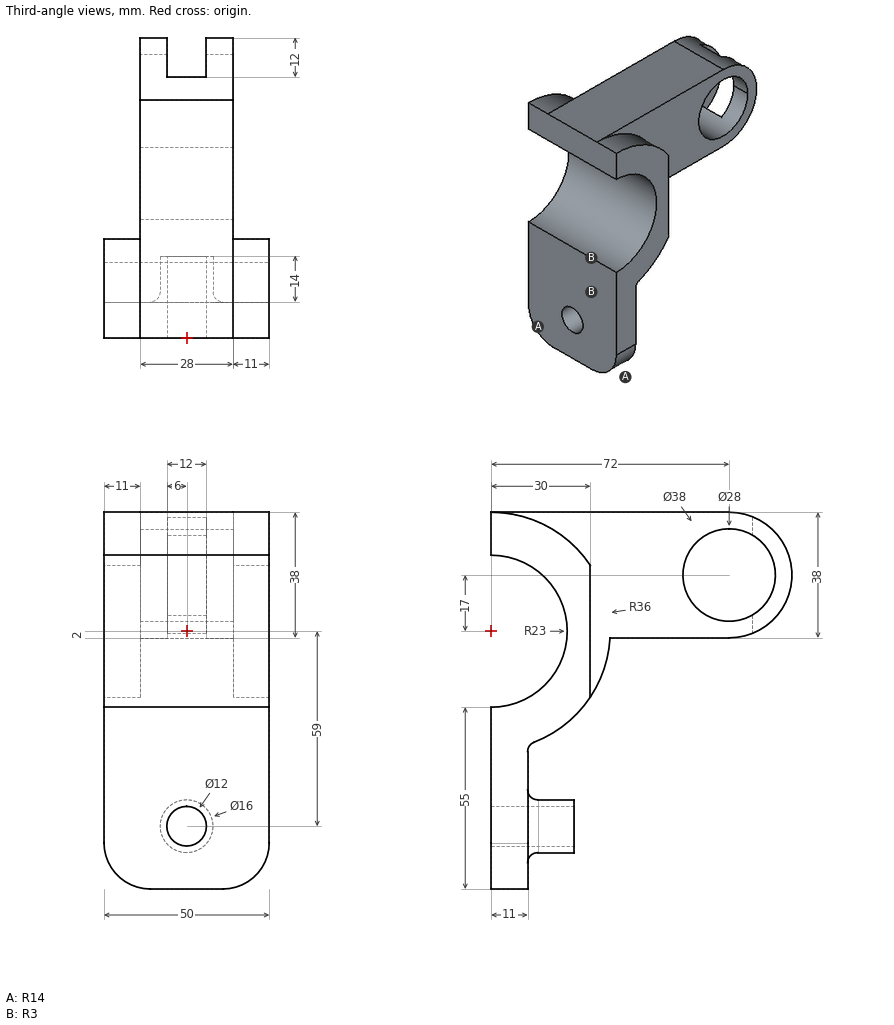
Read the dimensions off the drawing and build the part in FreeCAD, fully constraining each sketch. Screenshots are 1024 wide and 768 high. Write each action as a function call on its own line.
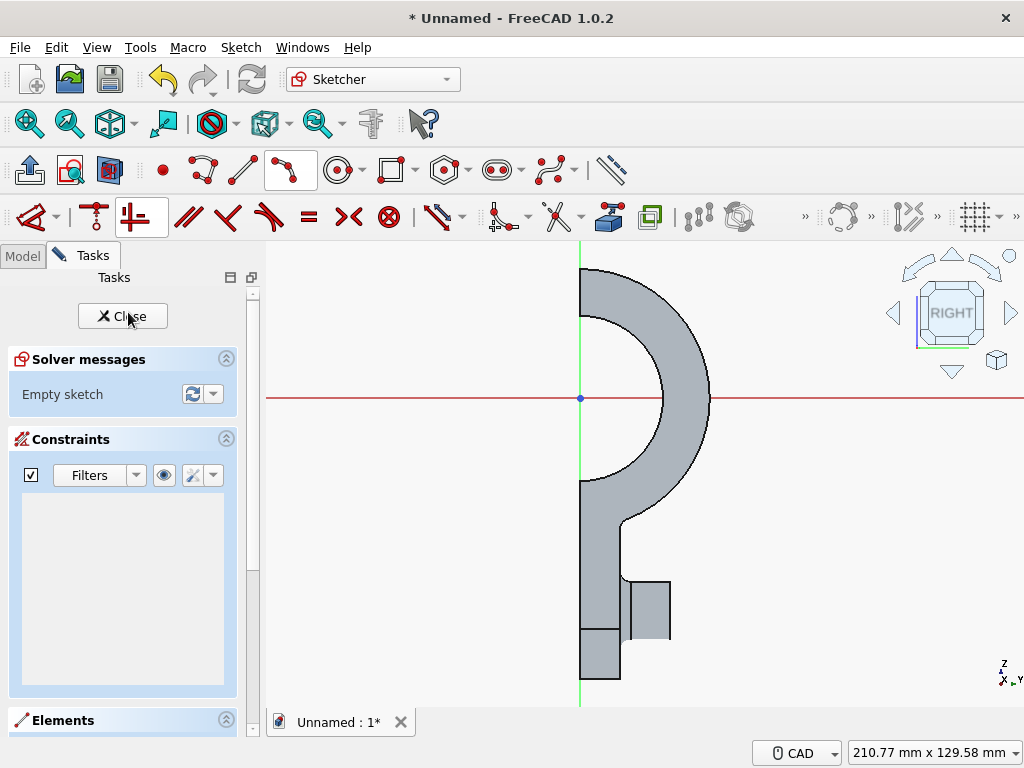
click(110, 170)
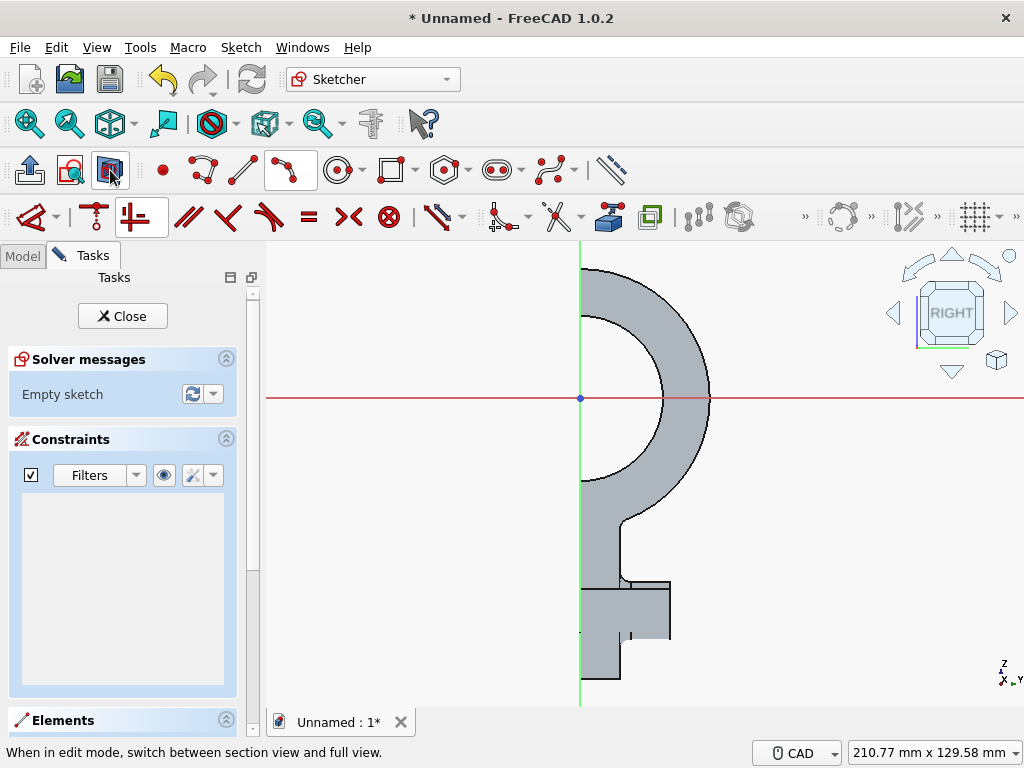
scroll(294, 679, down, 1)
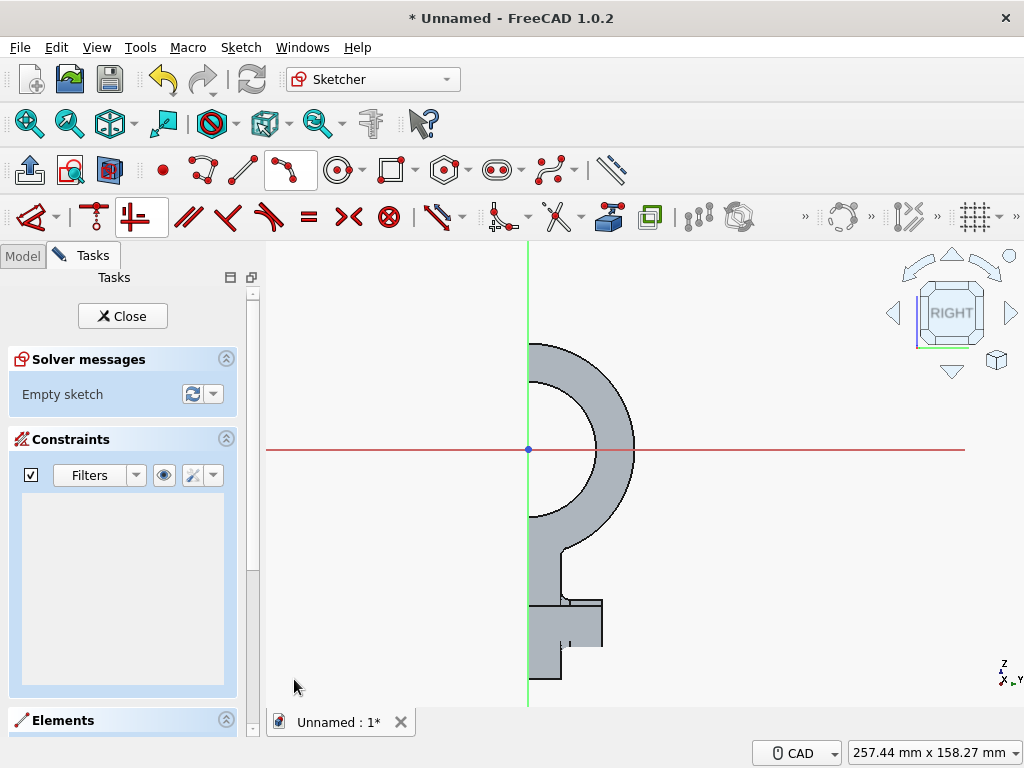
scroll(705, 309, up, 3)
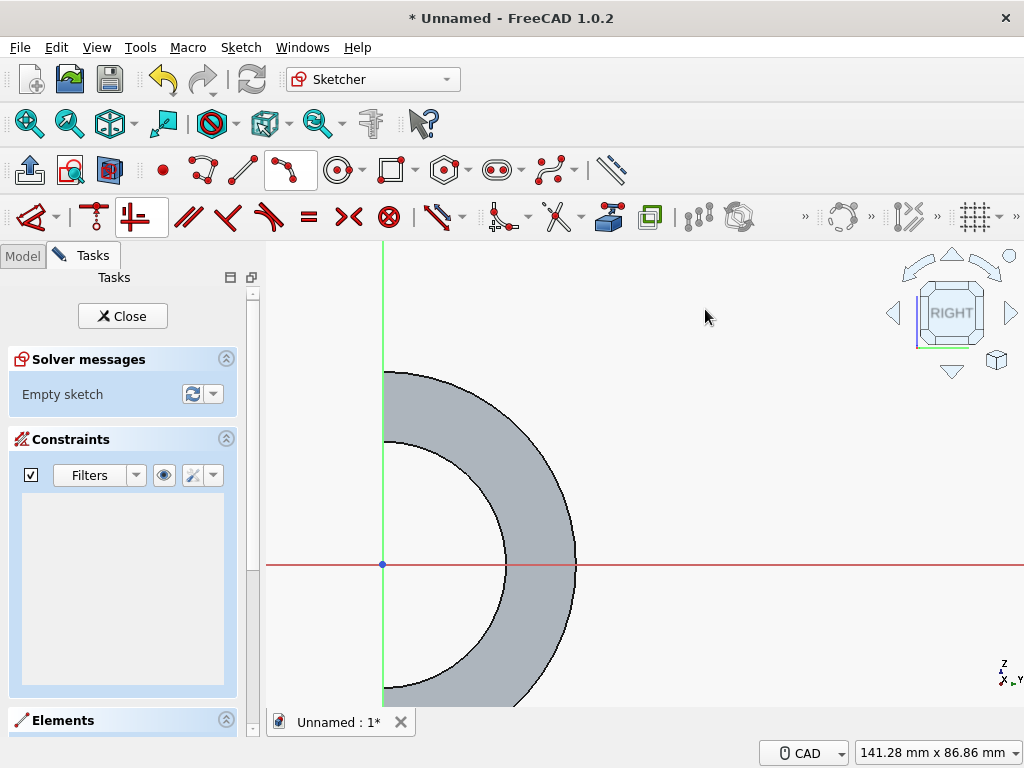
click(204, 170)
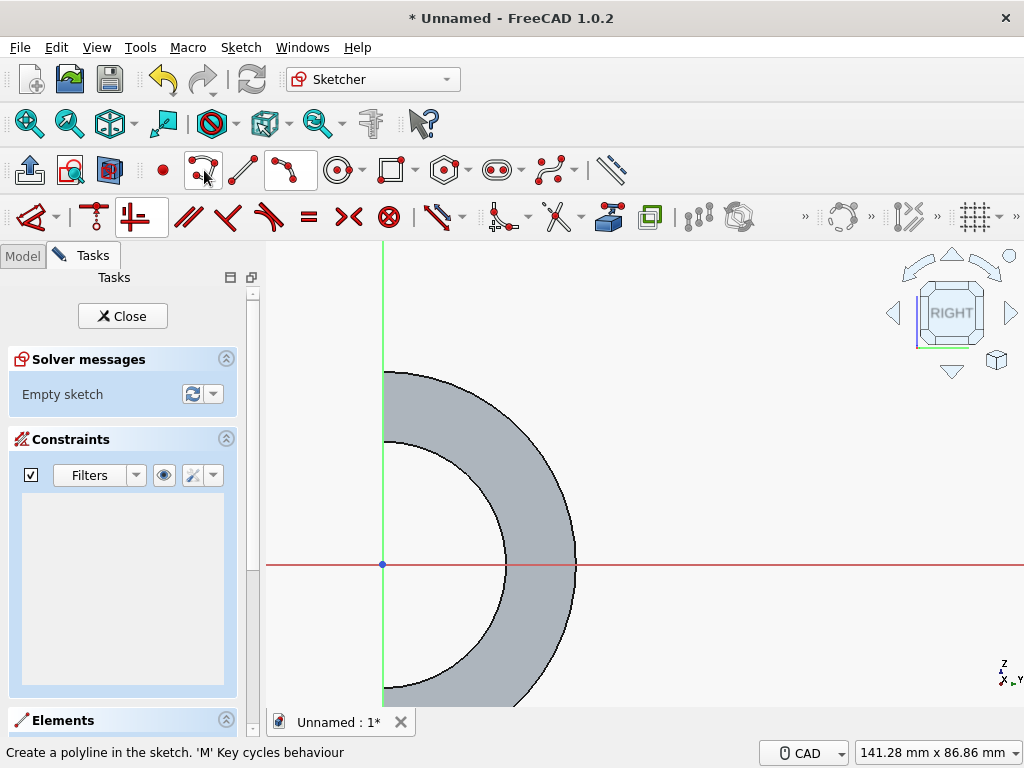
scroll(576, 576, up, 2)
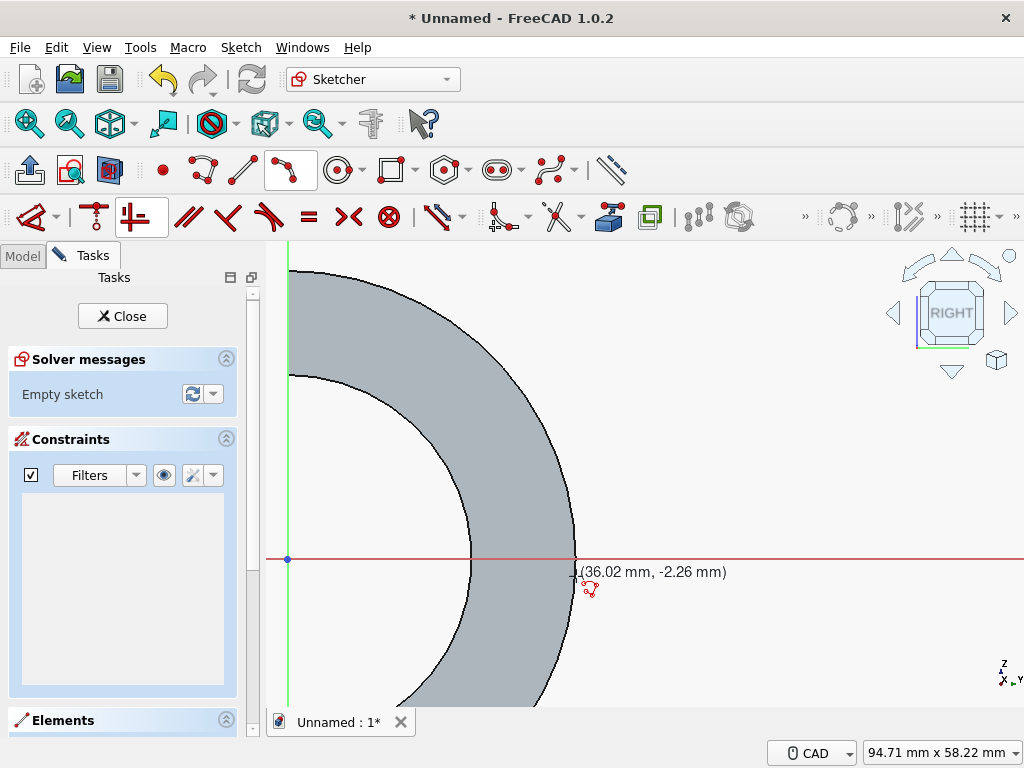
click(575, 575)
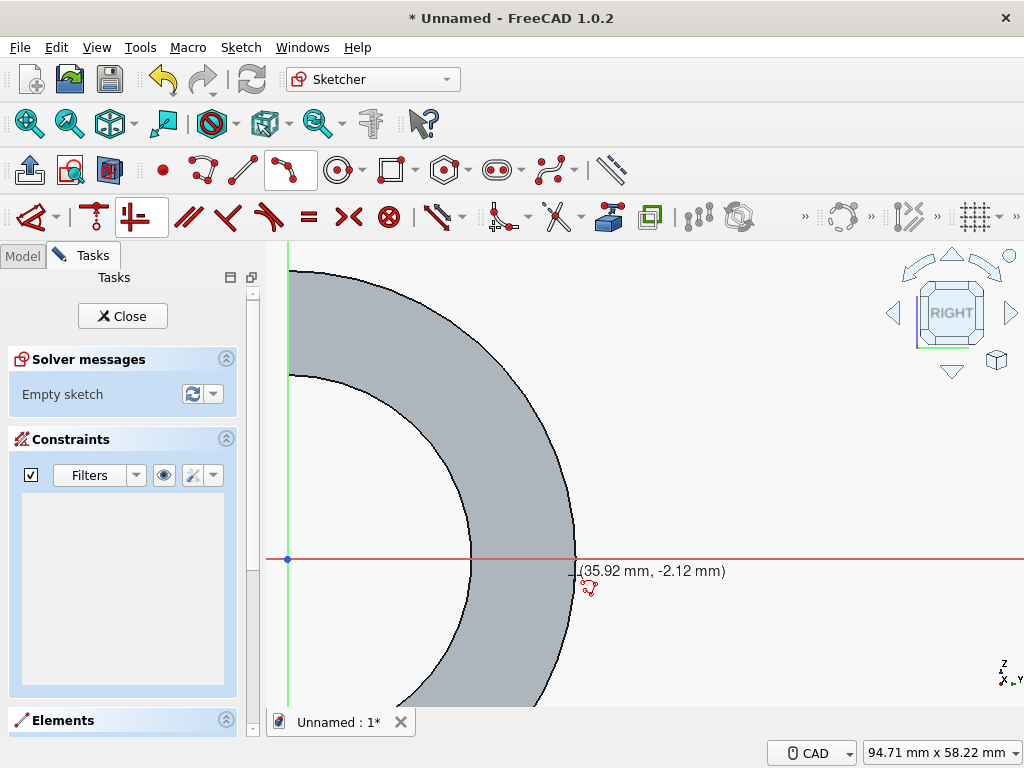
scroll(578, 578, down, 2)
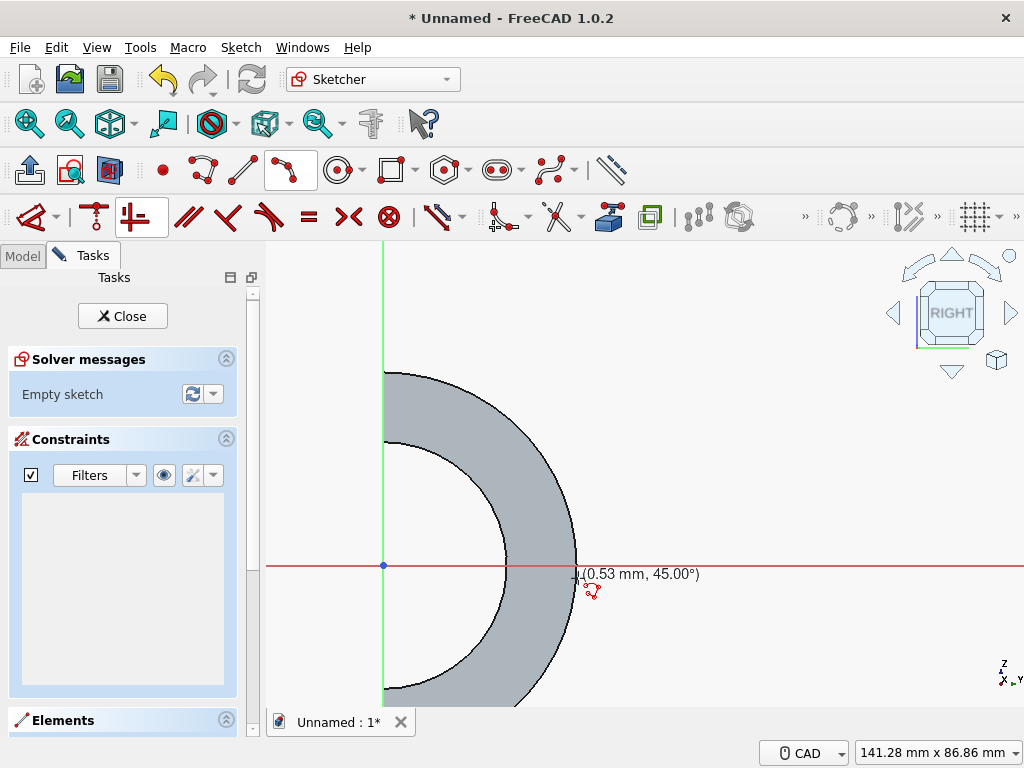
scroll(770, 576, up, 2)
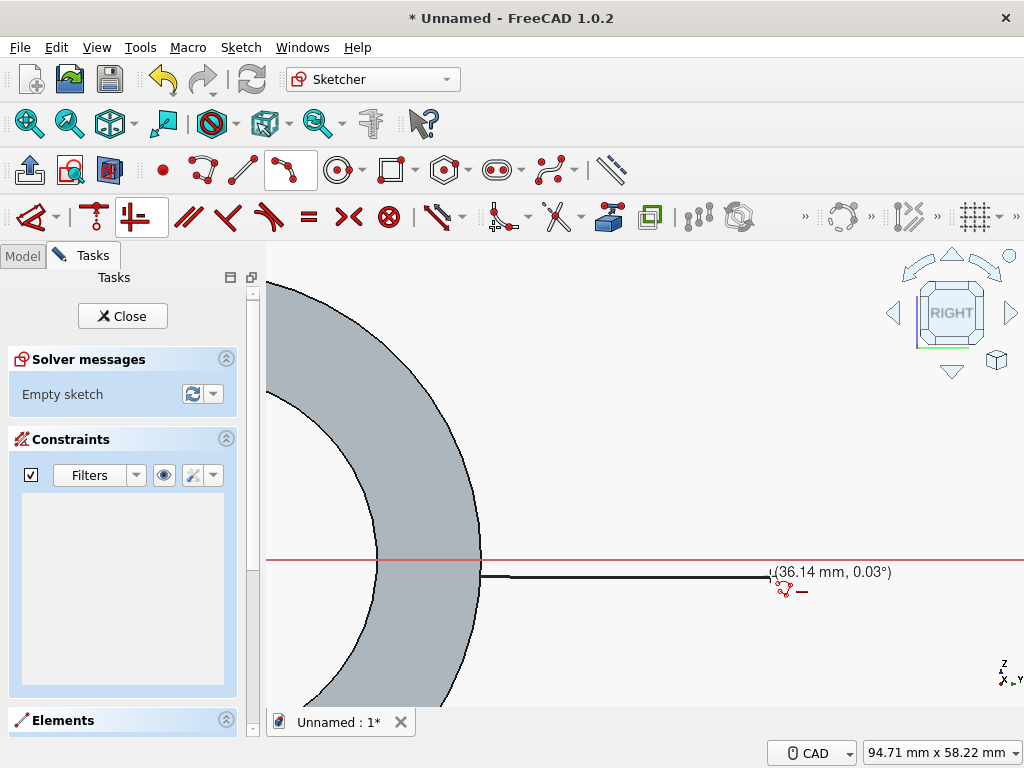
click(769, 576)
click(769, 272)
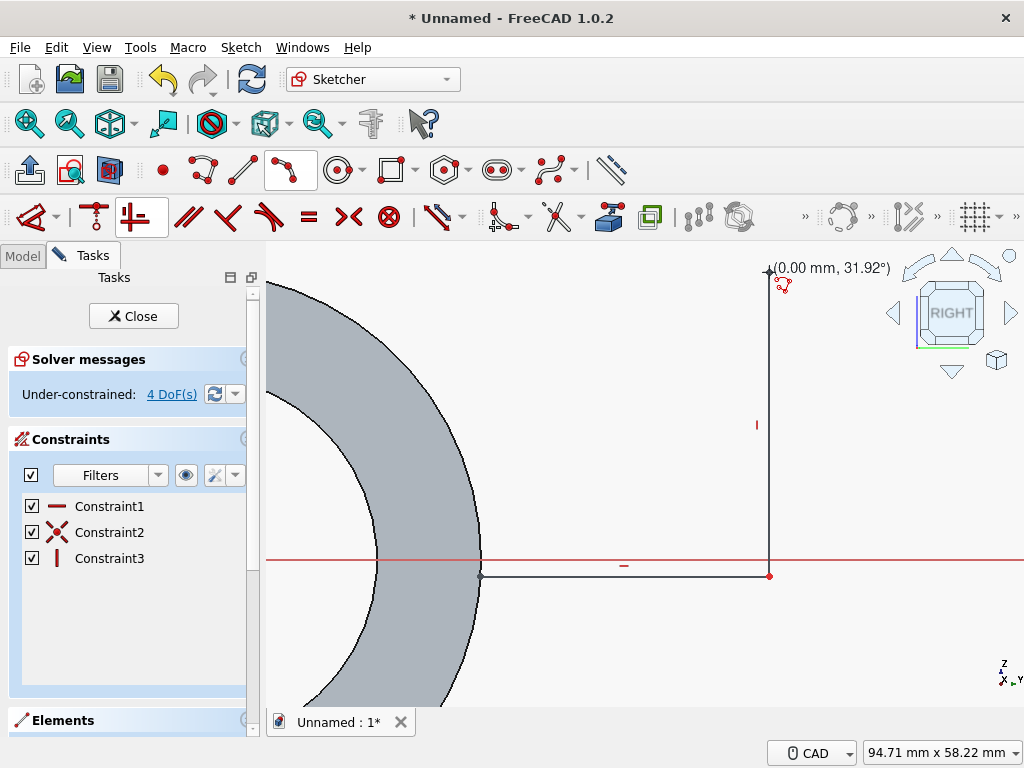
scroll(770, 576, down, 2)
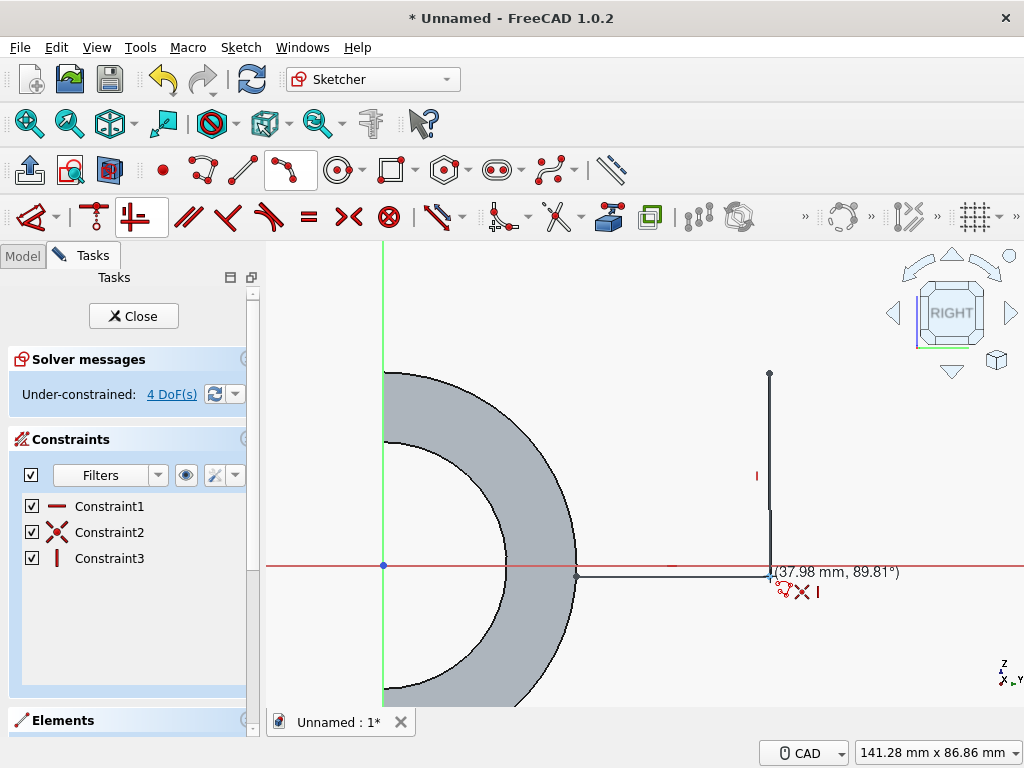
click(383, 372)
right_click(383, 372)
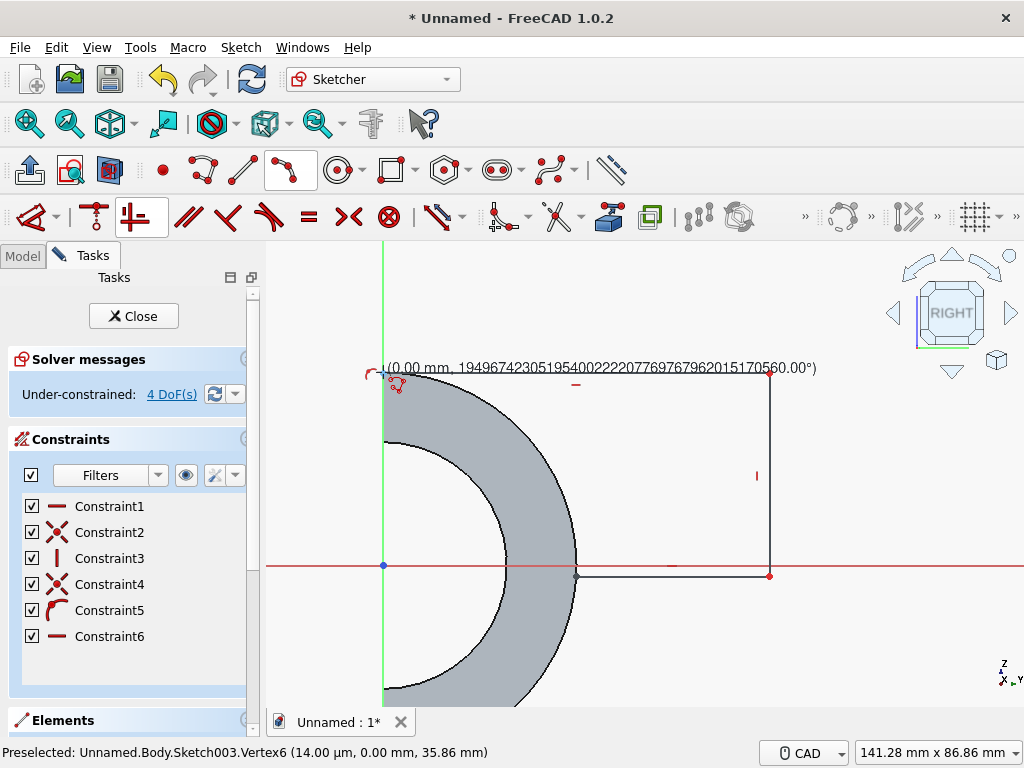
click(284, 170)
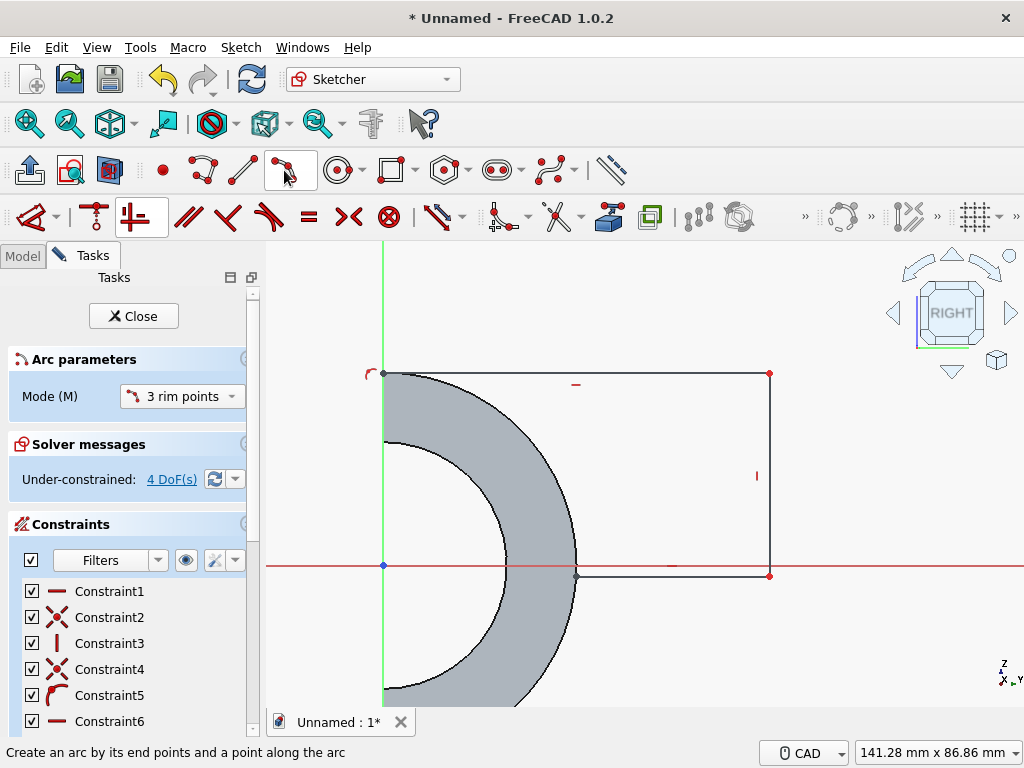
click(383, 373)